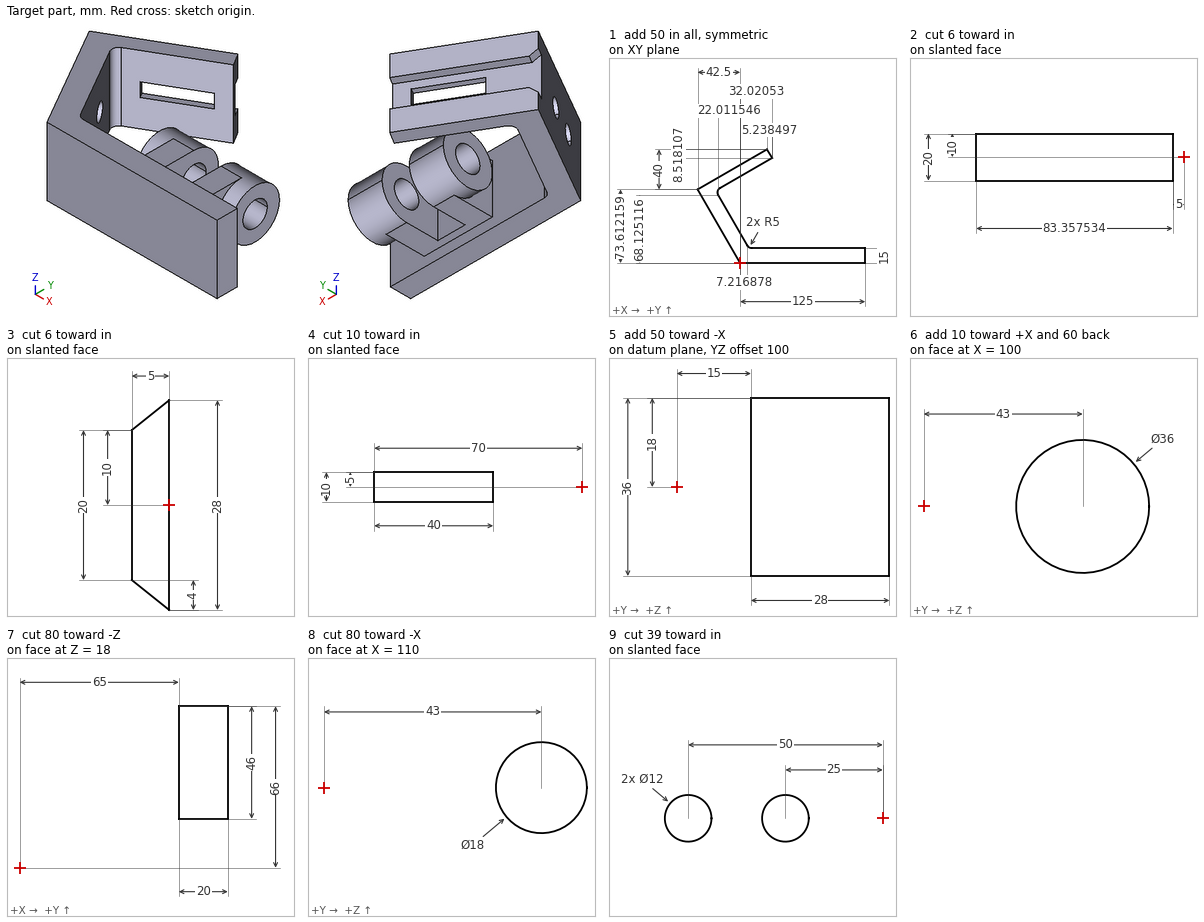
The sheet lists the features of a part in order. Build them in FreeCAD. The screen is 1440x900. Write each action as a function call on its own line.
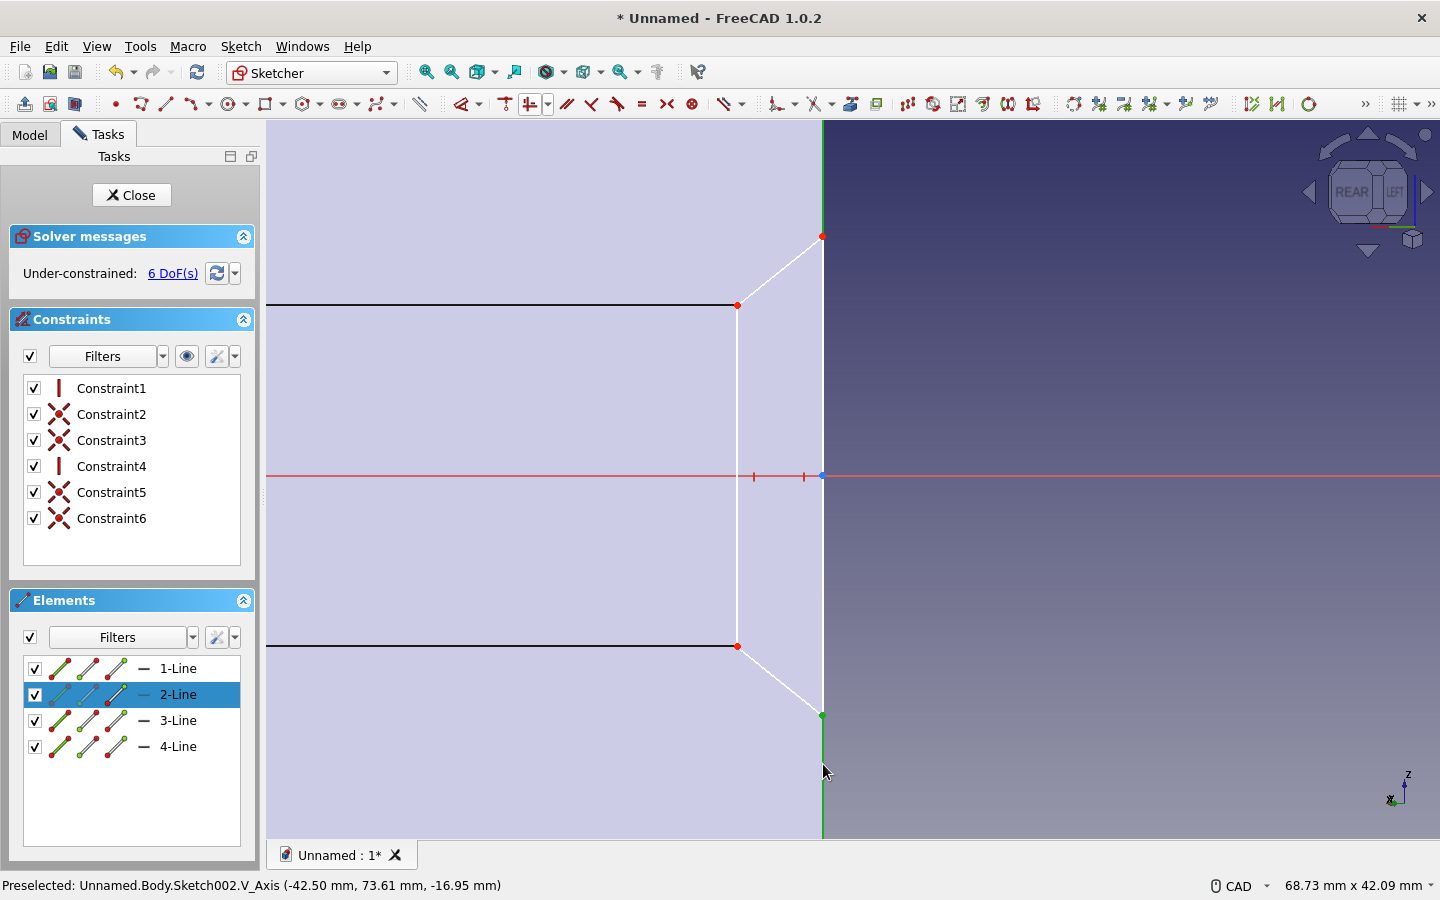
key(c)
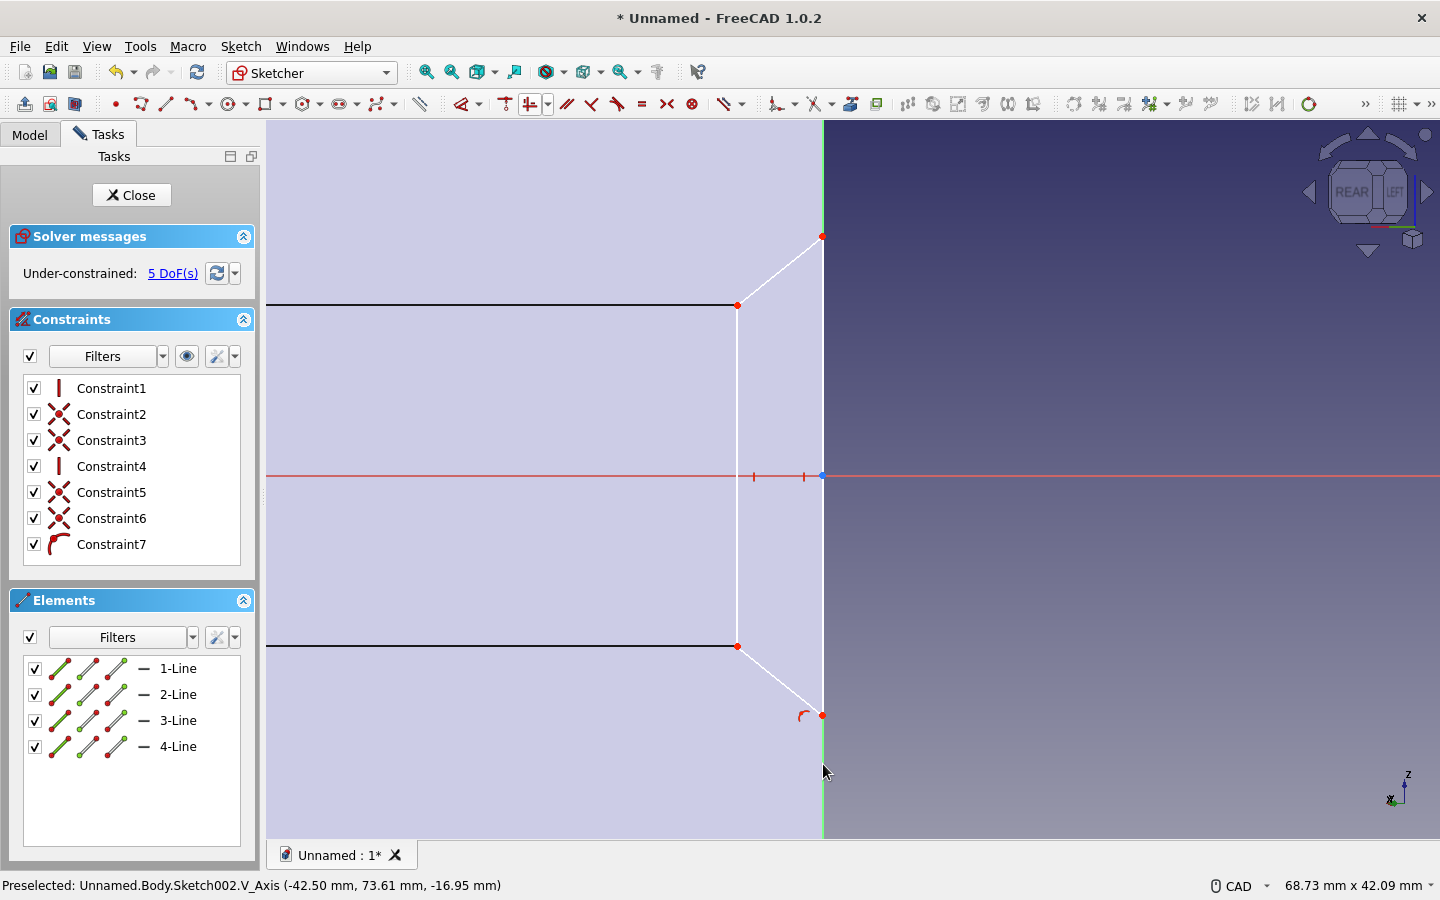
key(d)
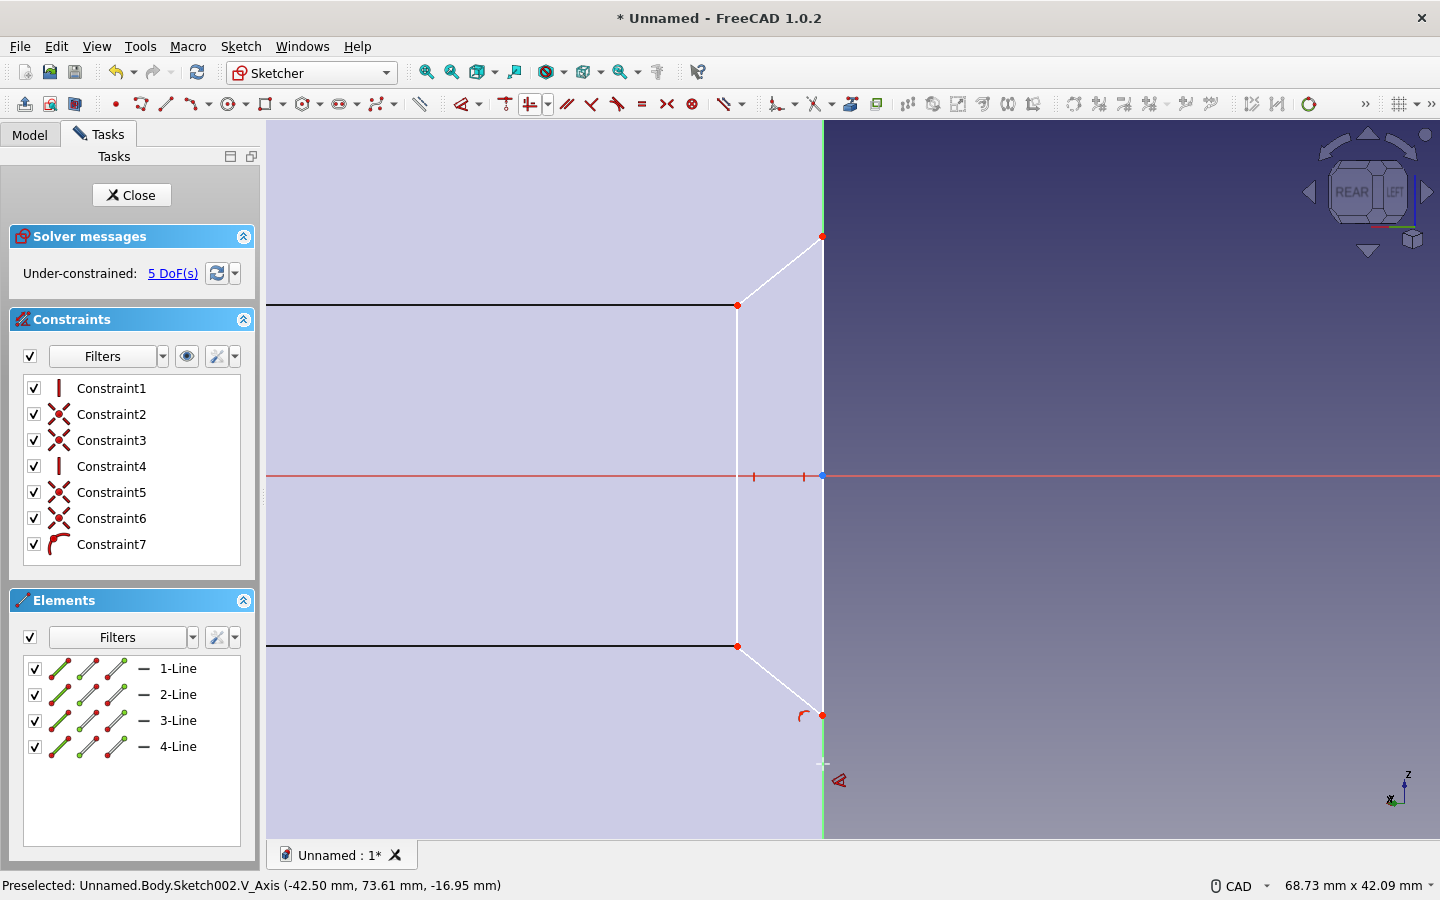
click(737, 408)
click(703, 398)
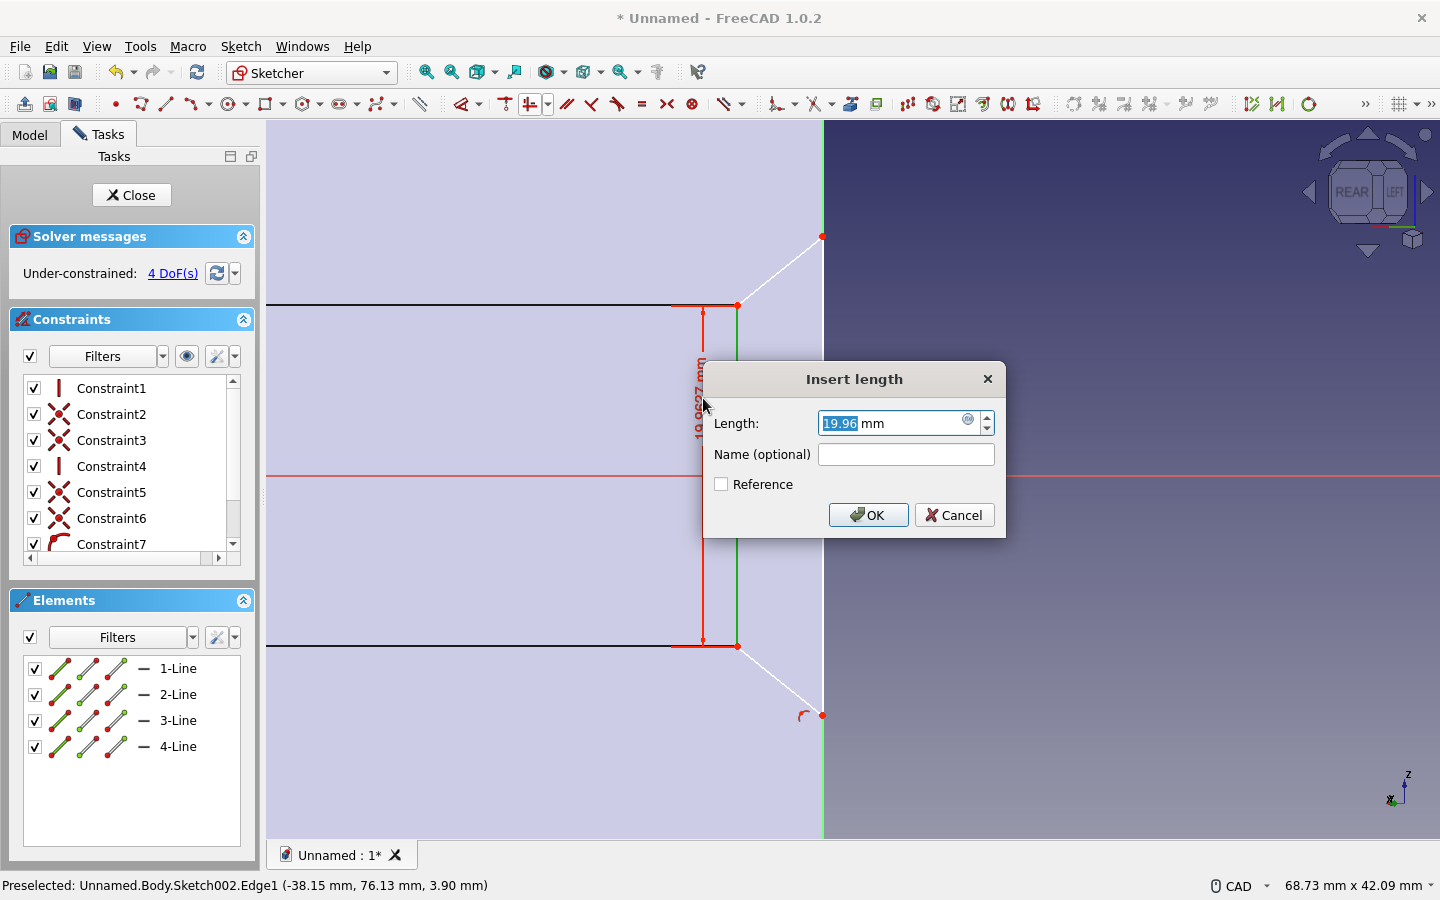
text(20)
key(Return)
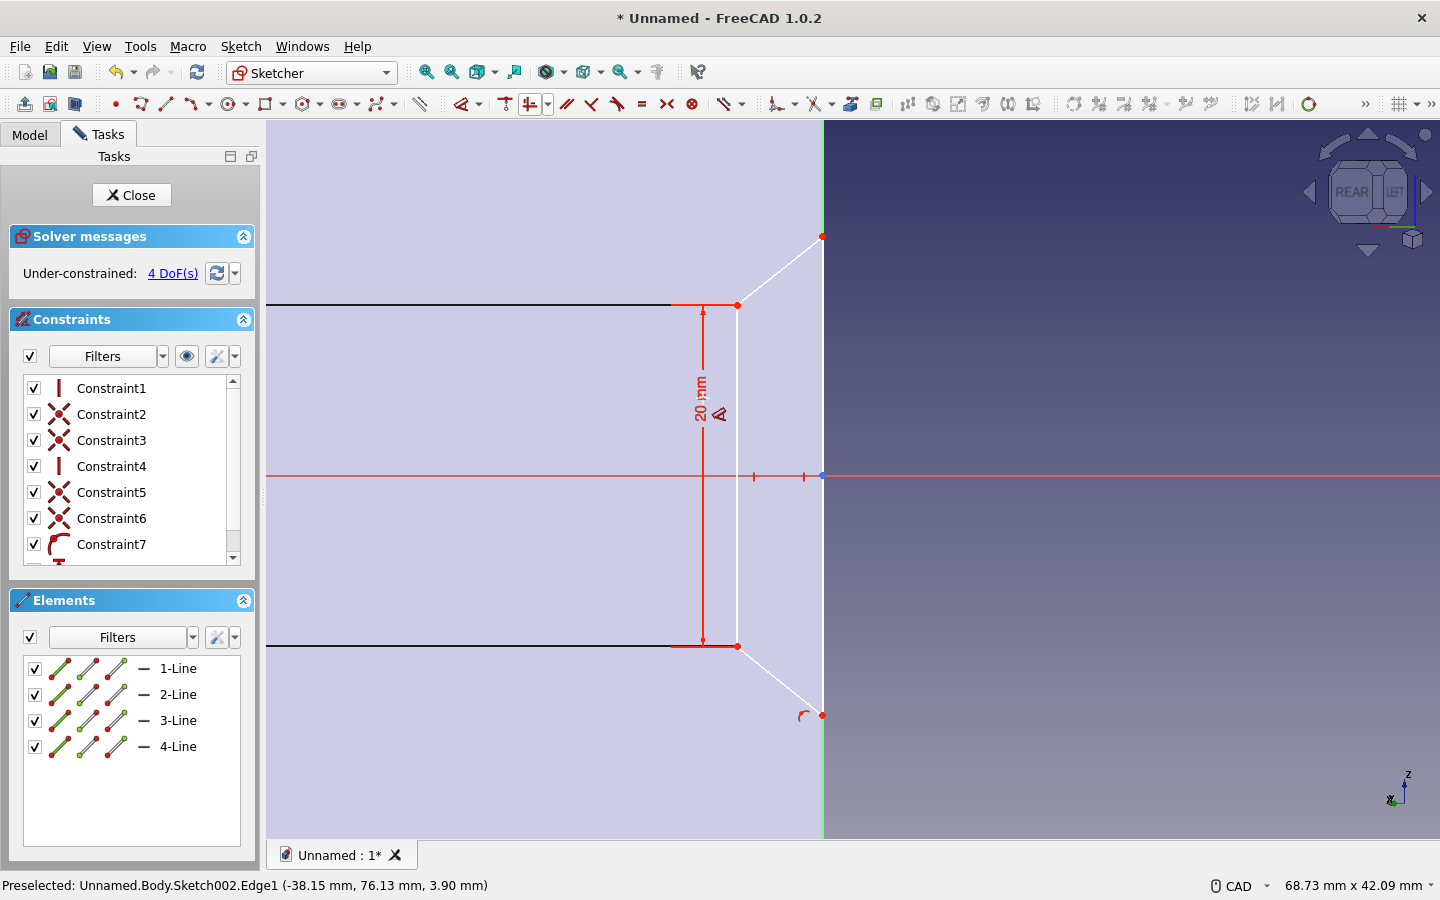
click(823, 572)
click(857, 366)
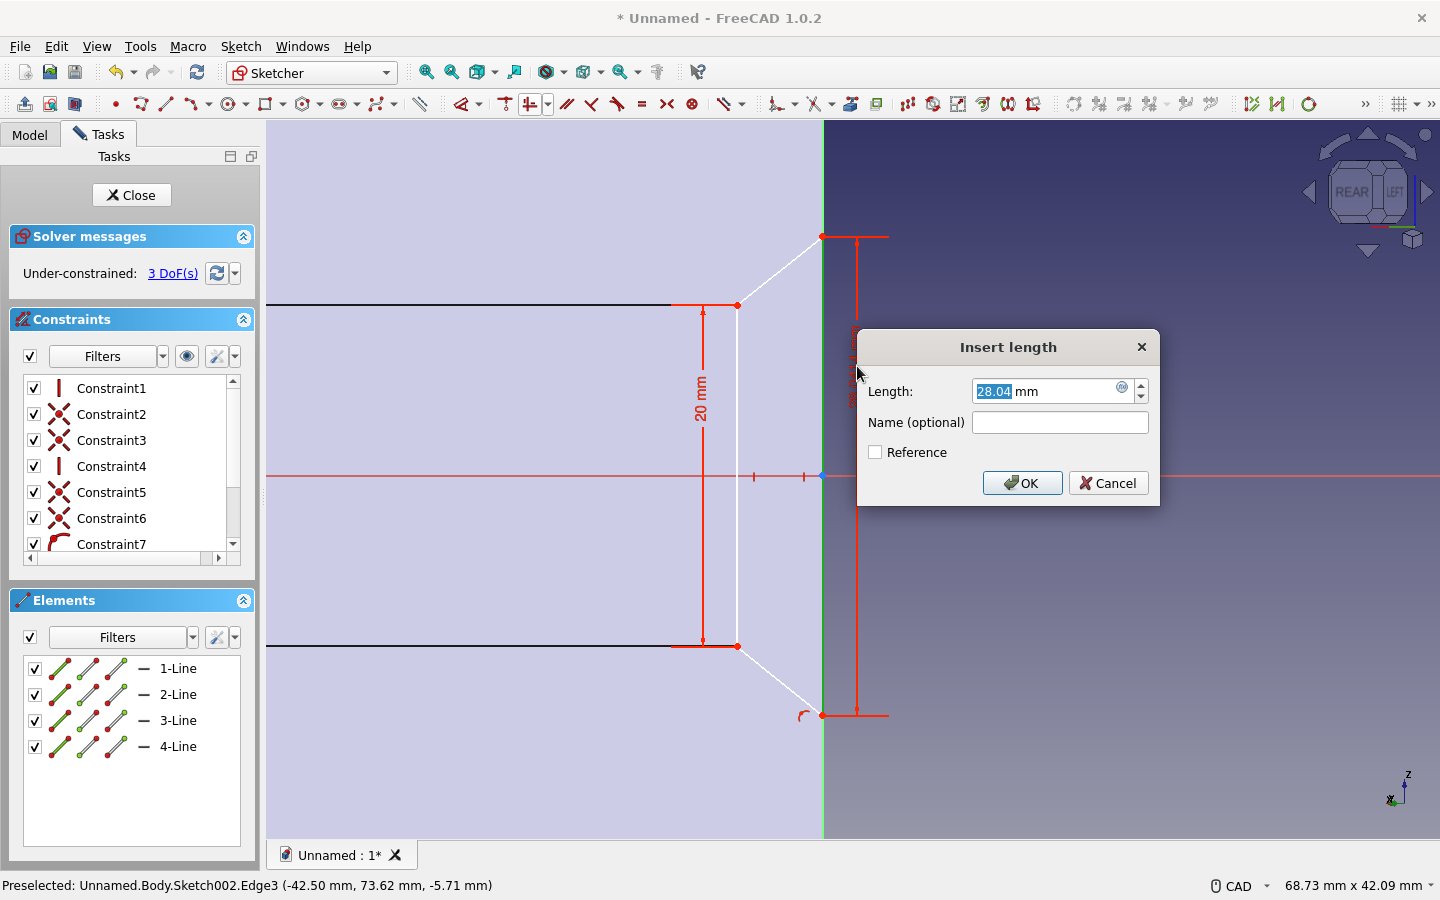
text(28)
key(Return)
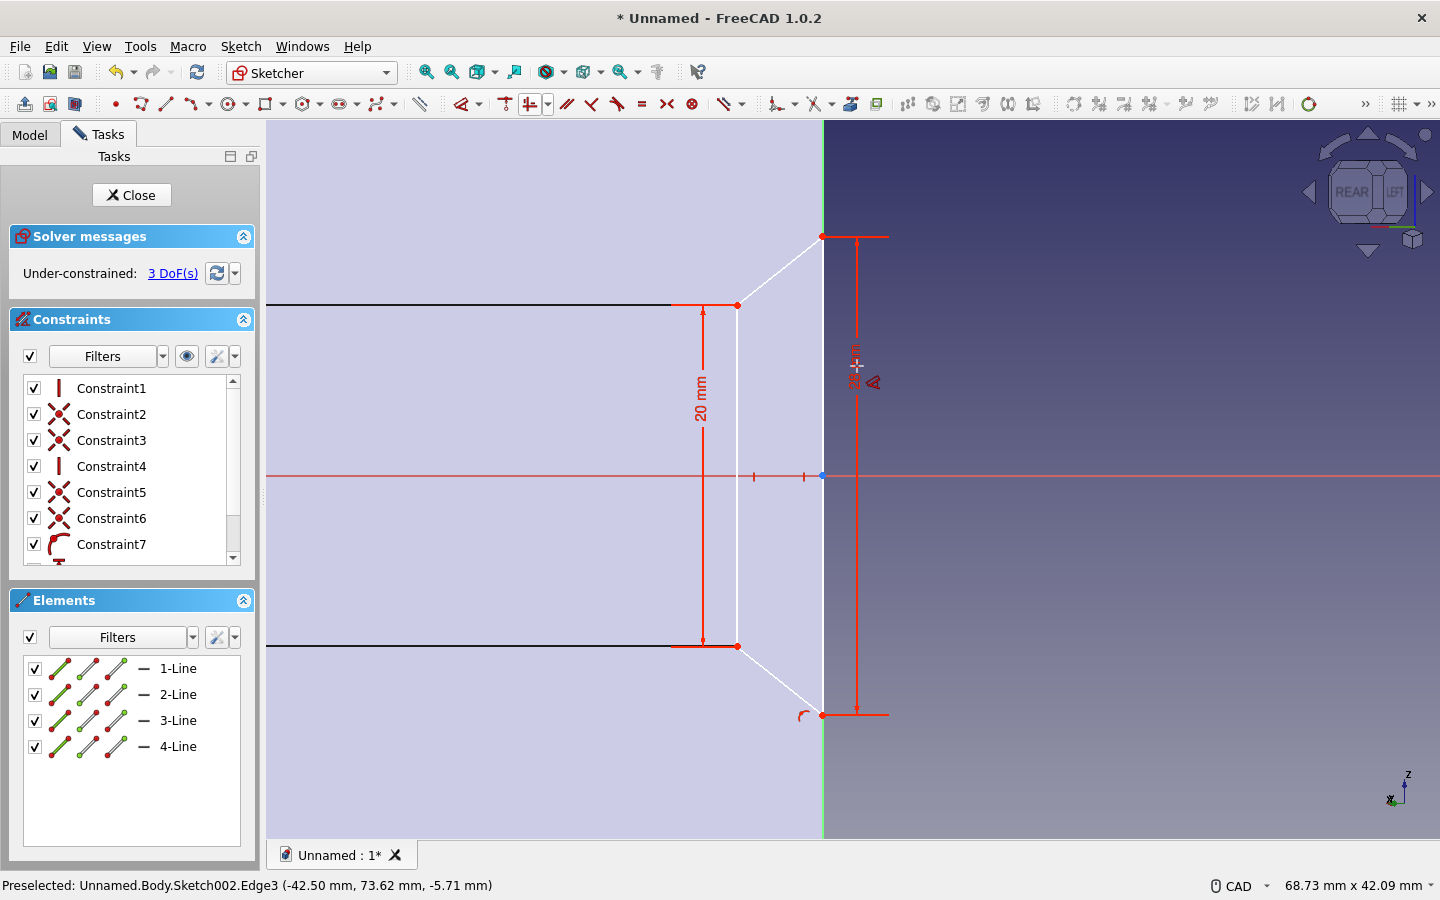
click(737, 305)
click(750, 271)